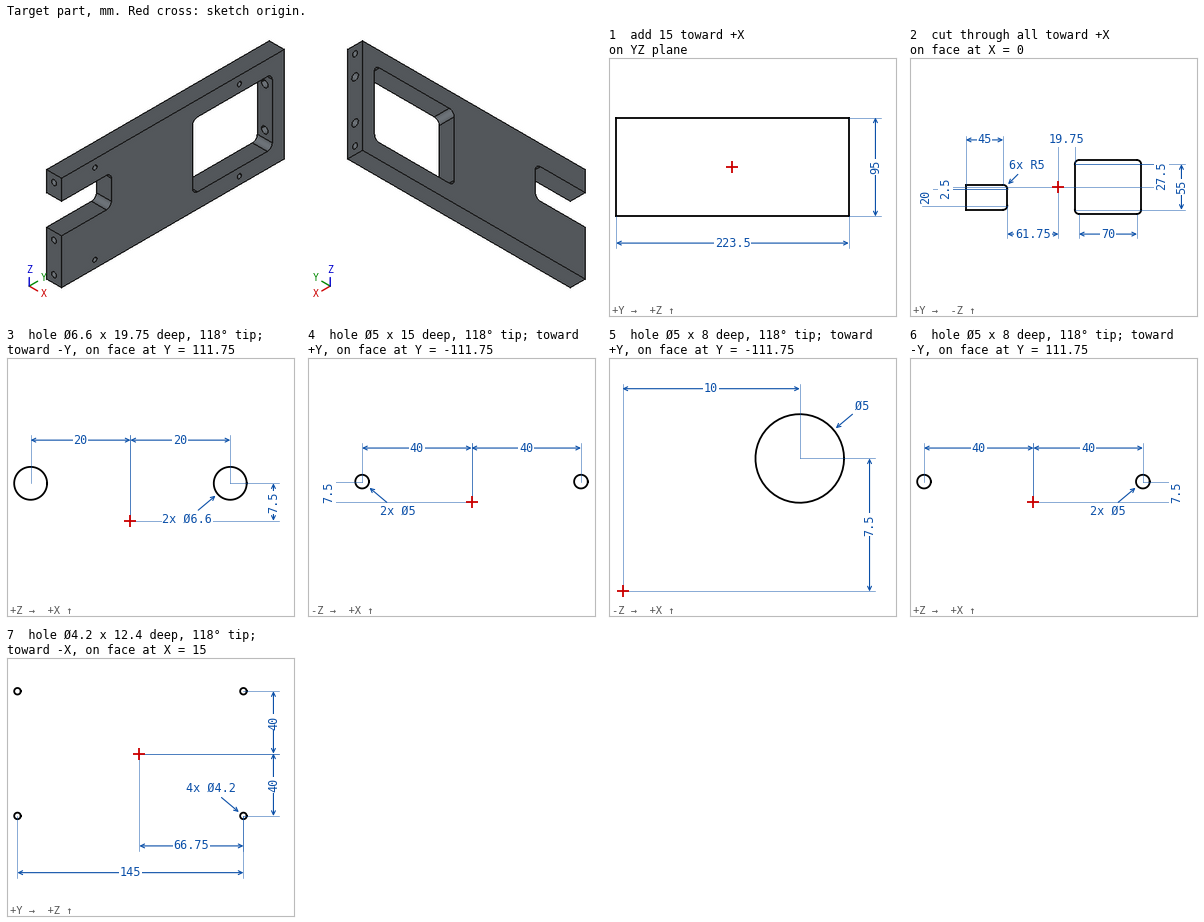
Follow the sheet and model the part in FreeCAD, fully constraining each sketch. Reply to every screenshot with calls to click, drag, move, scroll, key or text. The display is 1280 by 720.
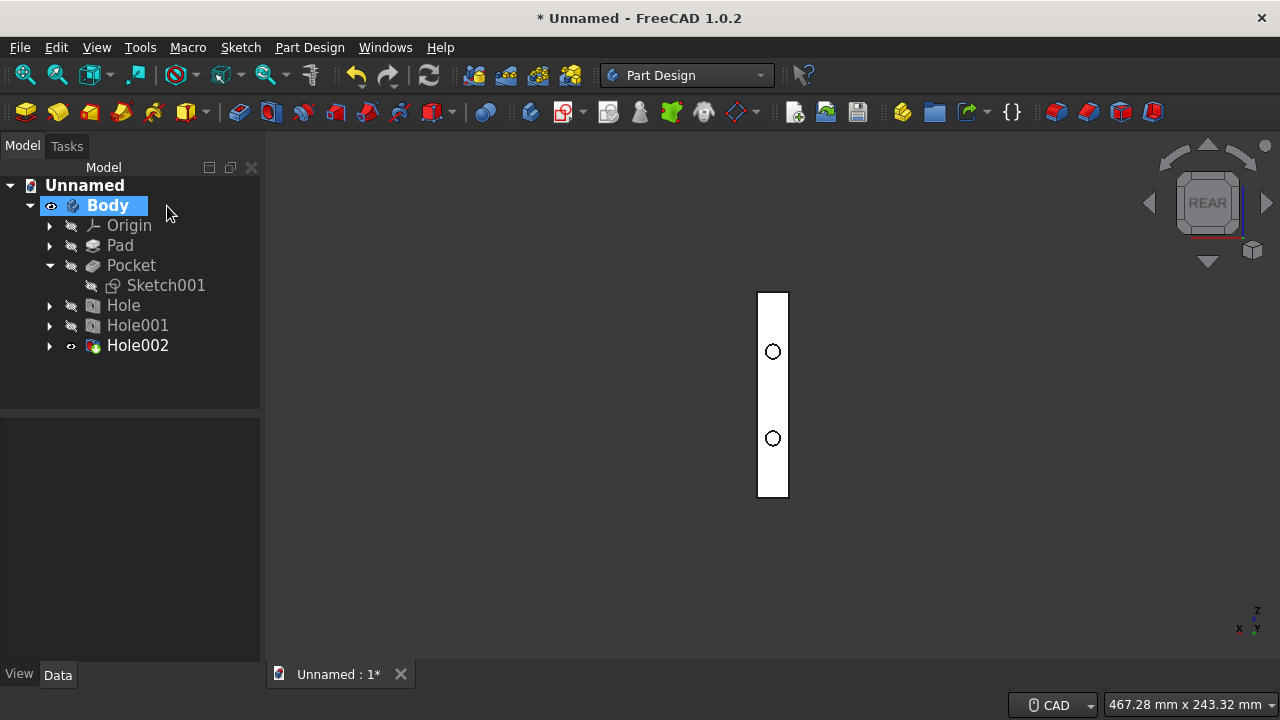
click(26, 76)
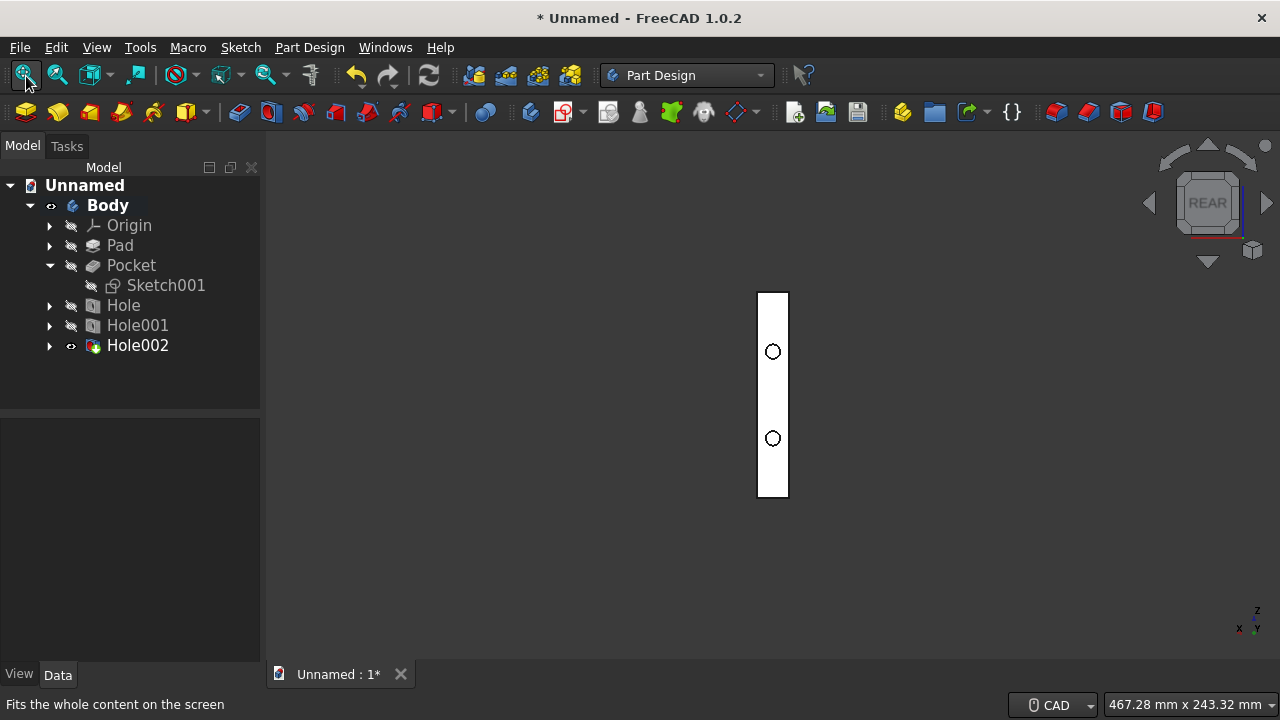
click(773, 394)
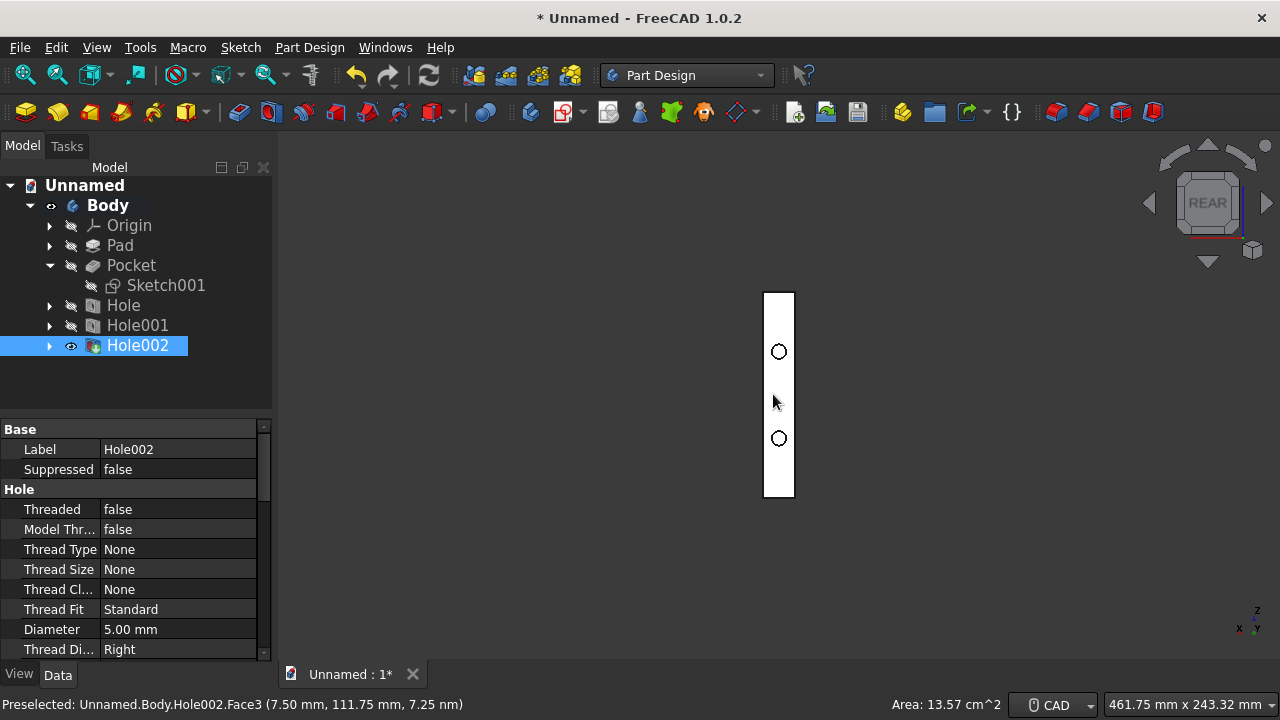
click(564, 112)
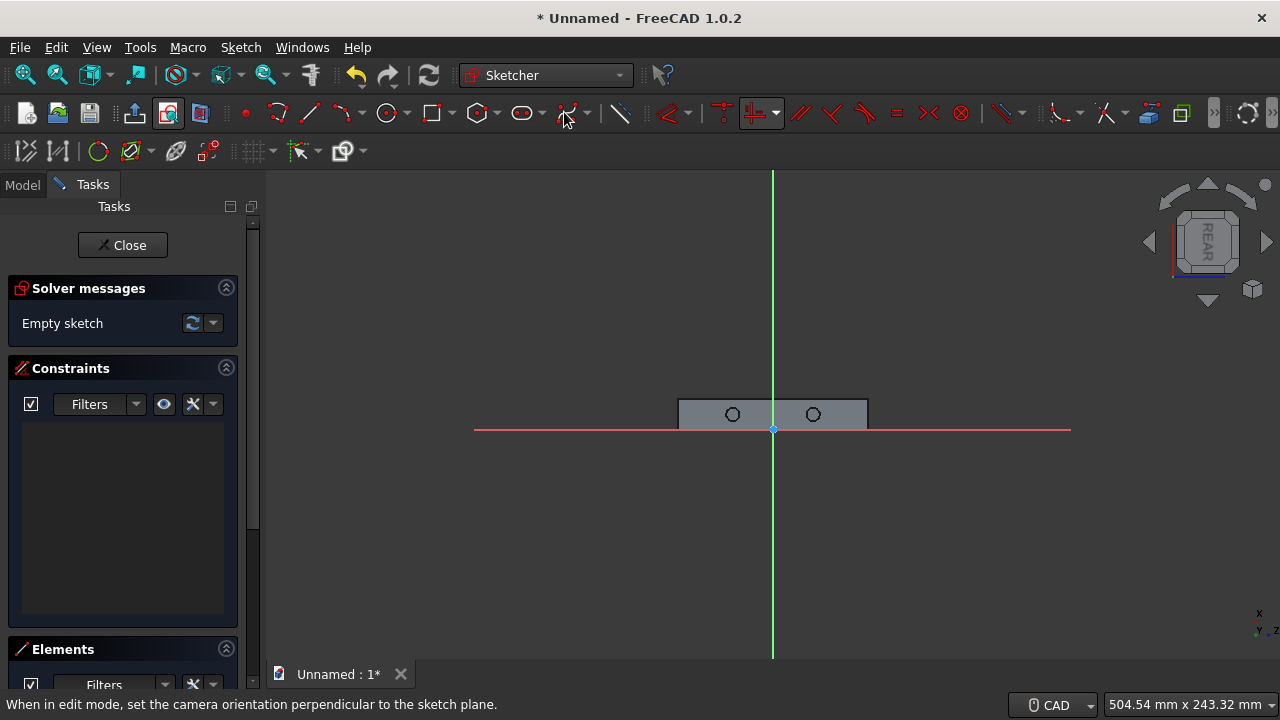
scroll(803, 422, up, 6)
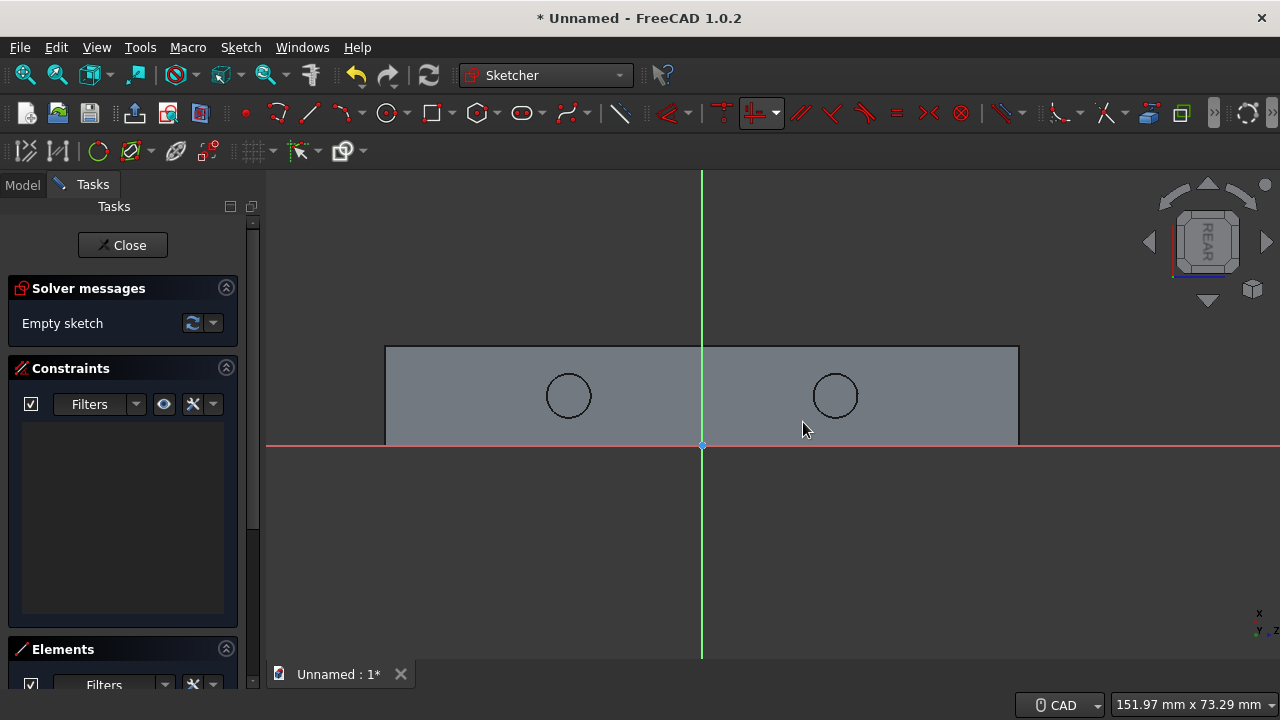
click(388, 114)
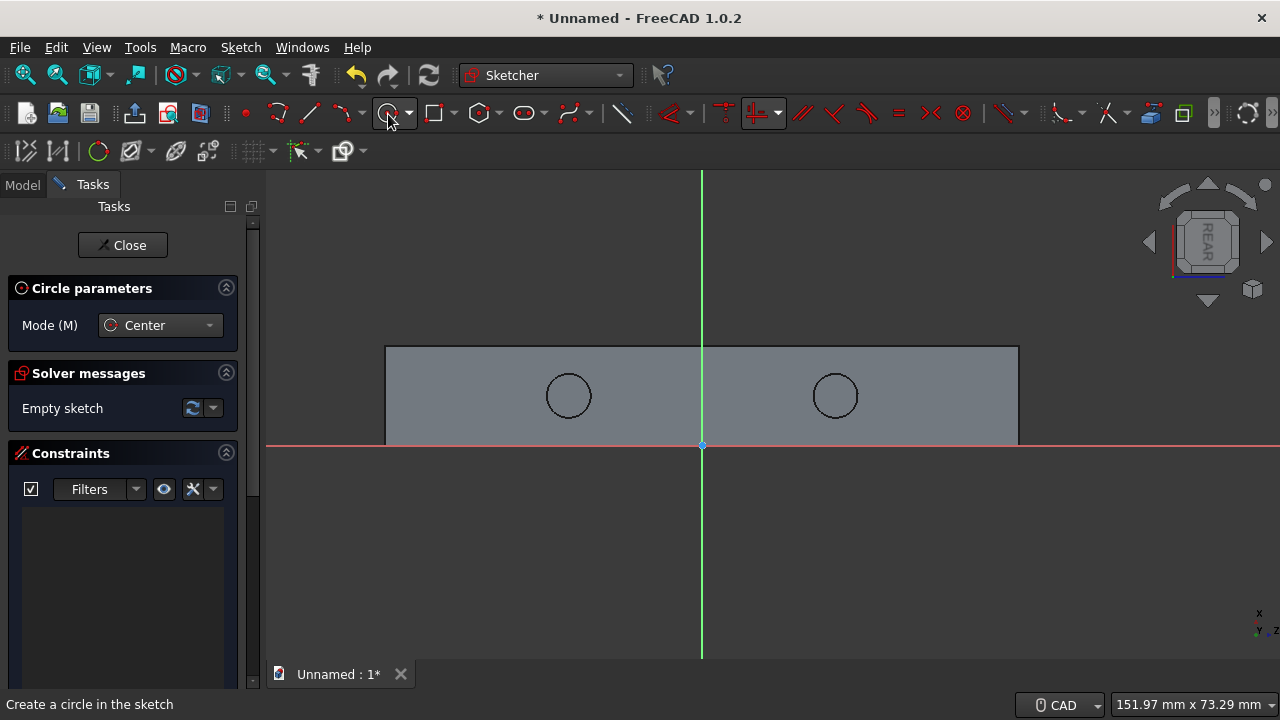
scroll(969, 396, up, 2)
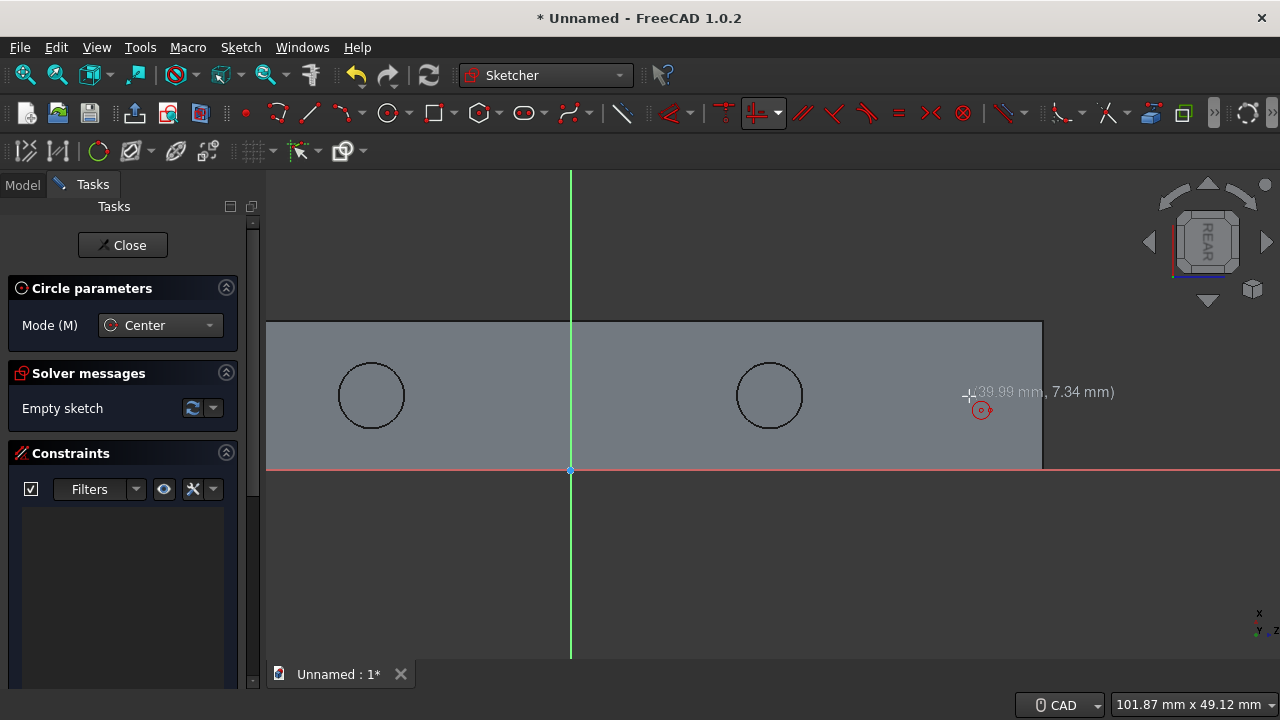
click(969, 396)
move(986, 378)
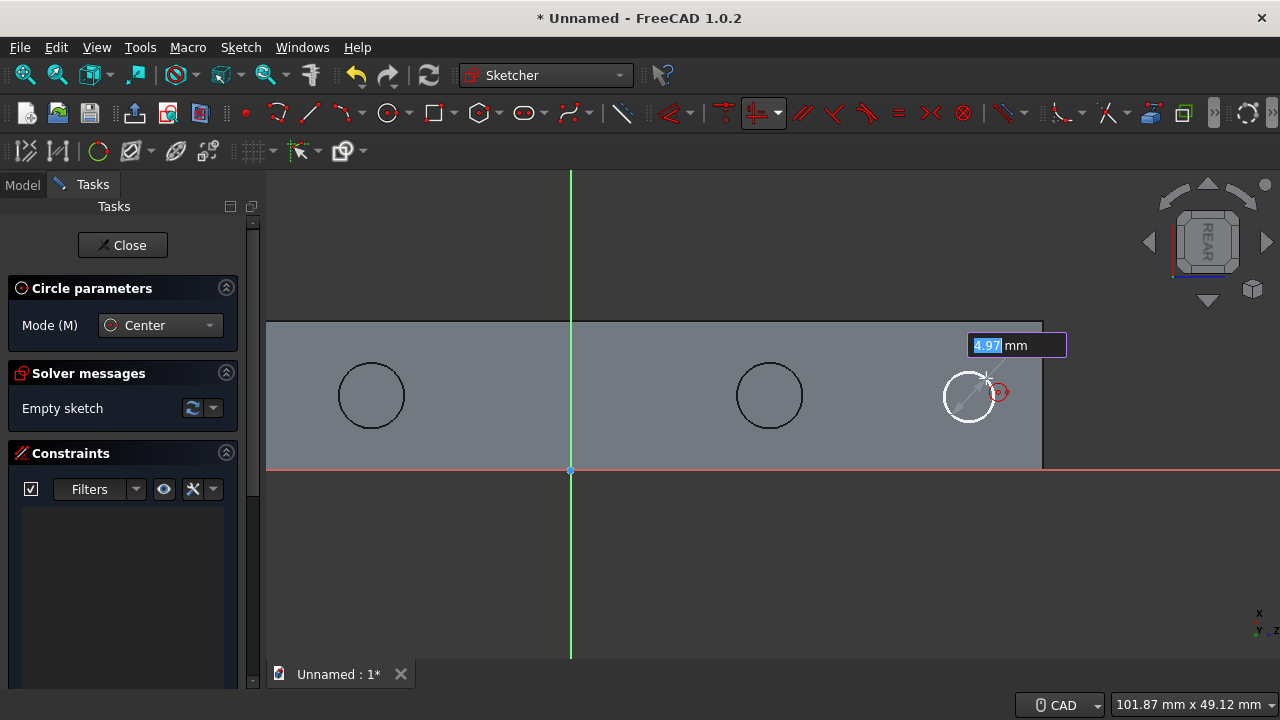
text(5)
key(Return)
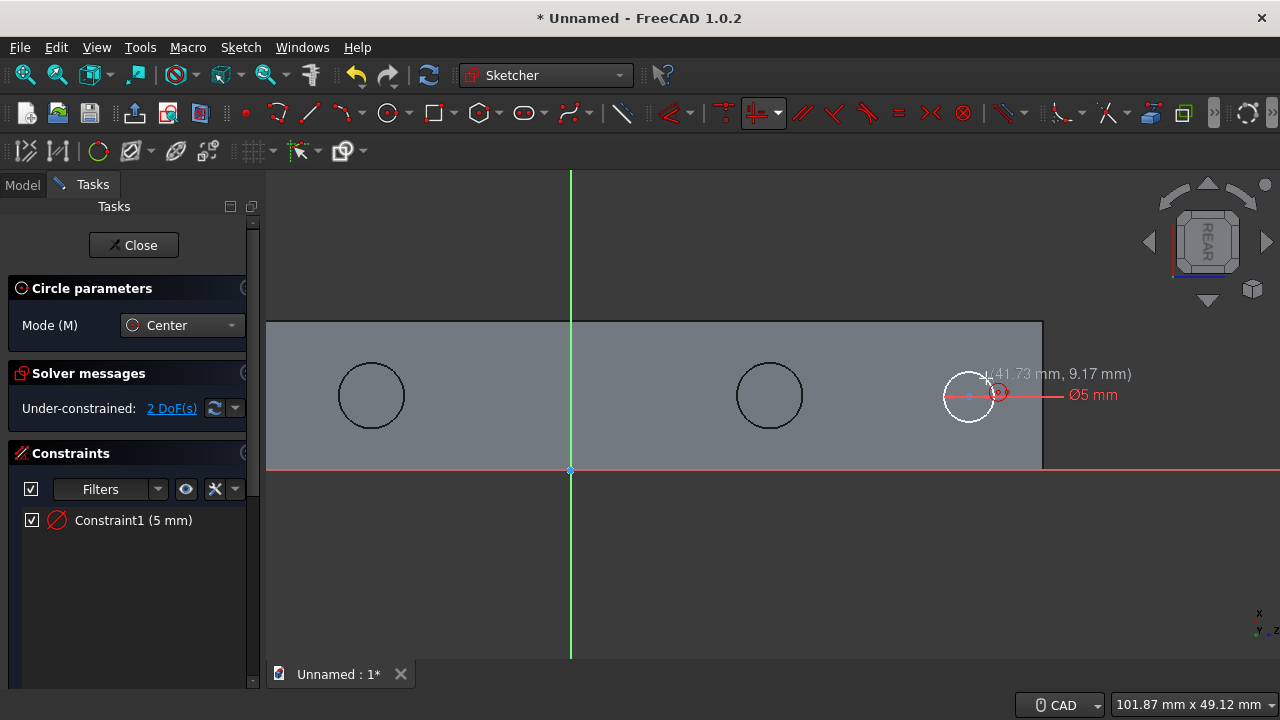
scroll(977, 402, down, 2)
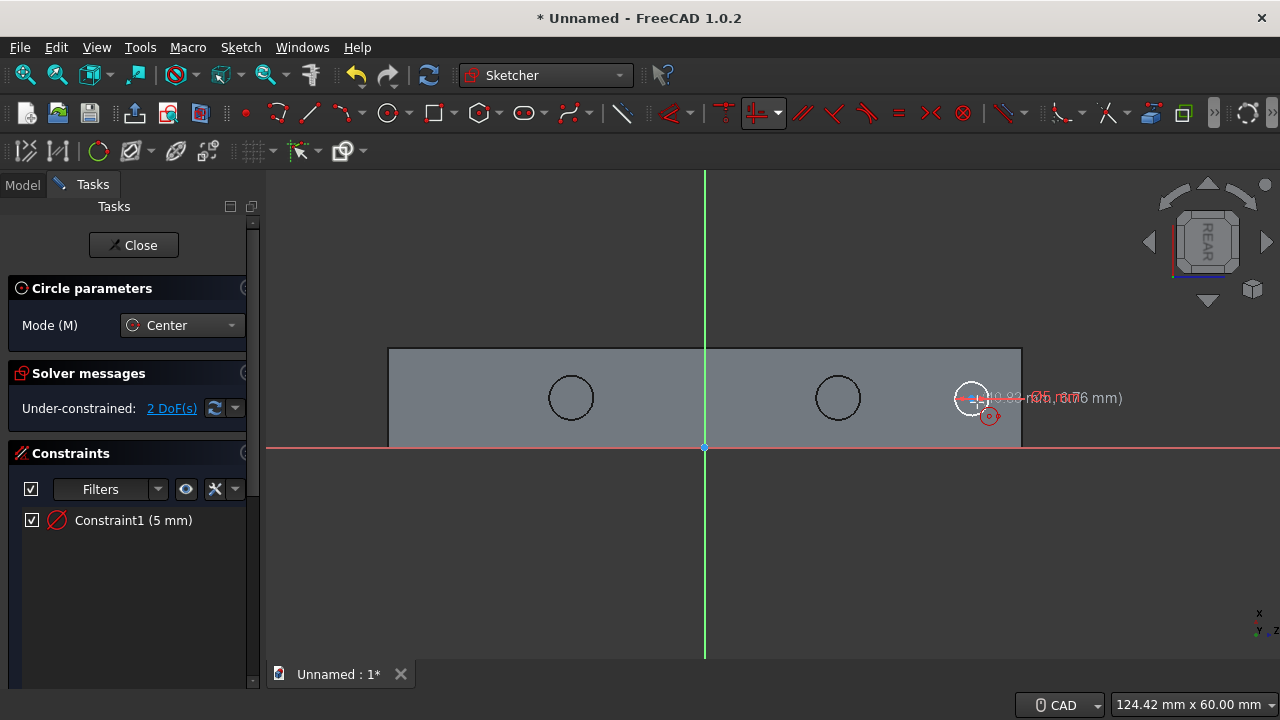
scroll(438, 398, up, 2)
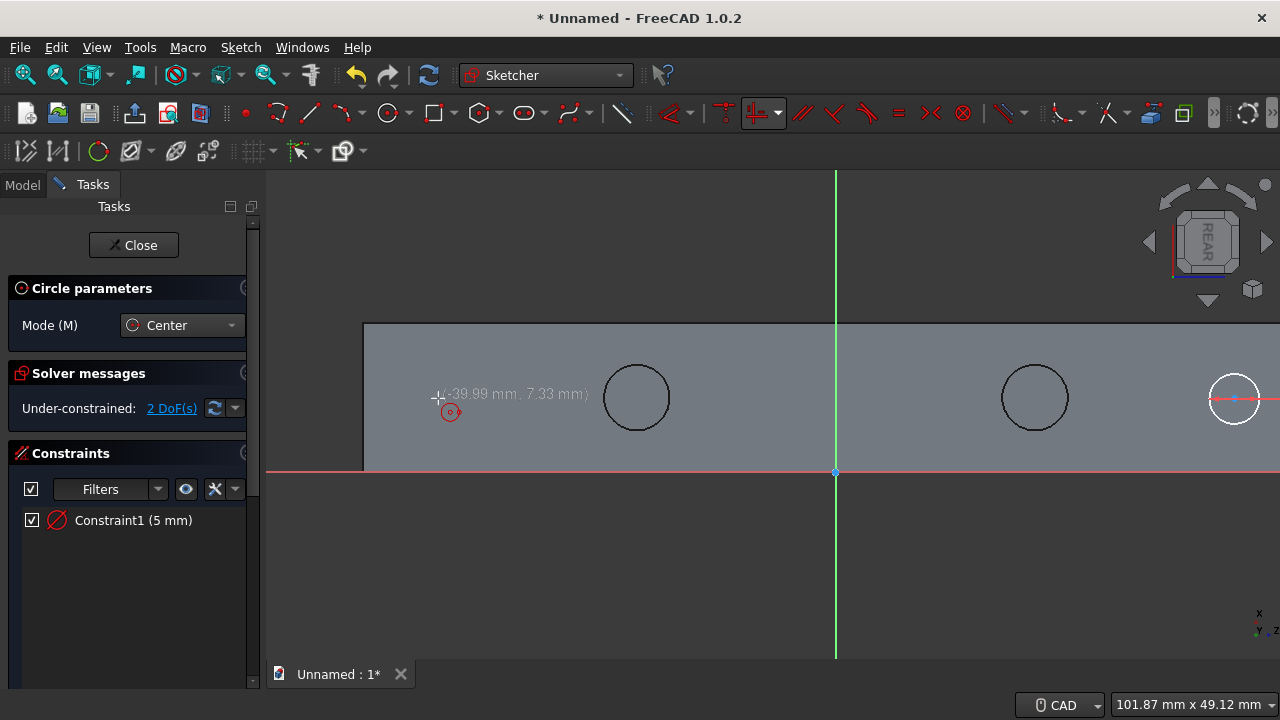
click(438, 398)
move(455, 380)